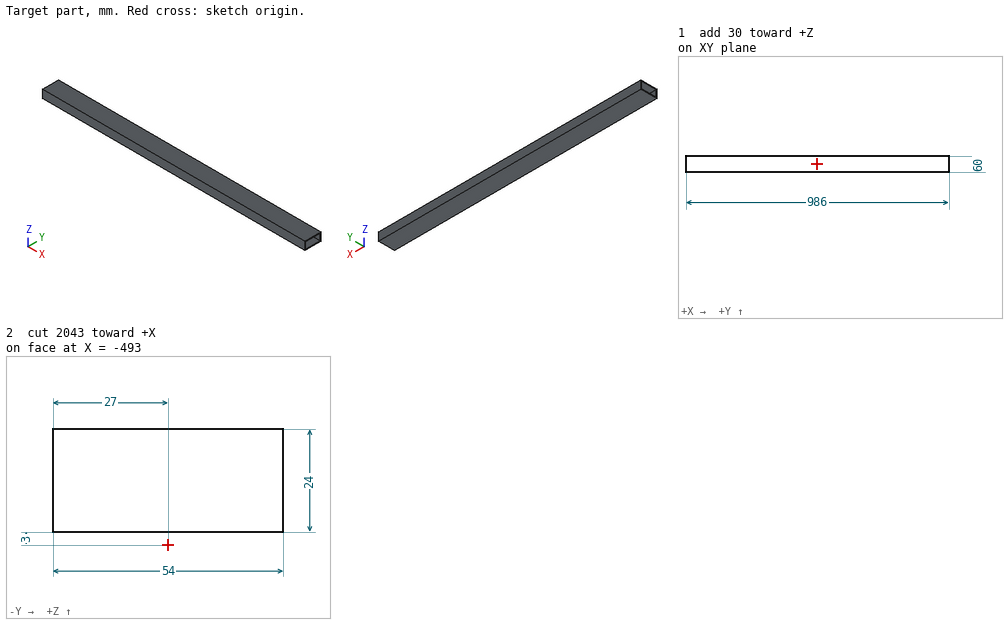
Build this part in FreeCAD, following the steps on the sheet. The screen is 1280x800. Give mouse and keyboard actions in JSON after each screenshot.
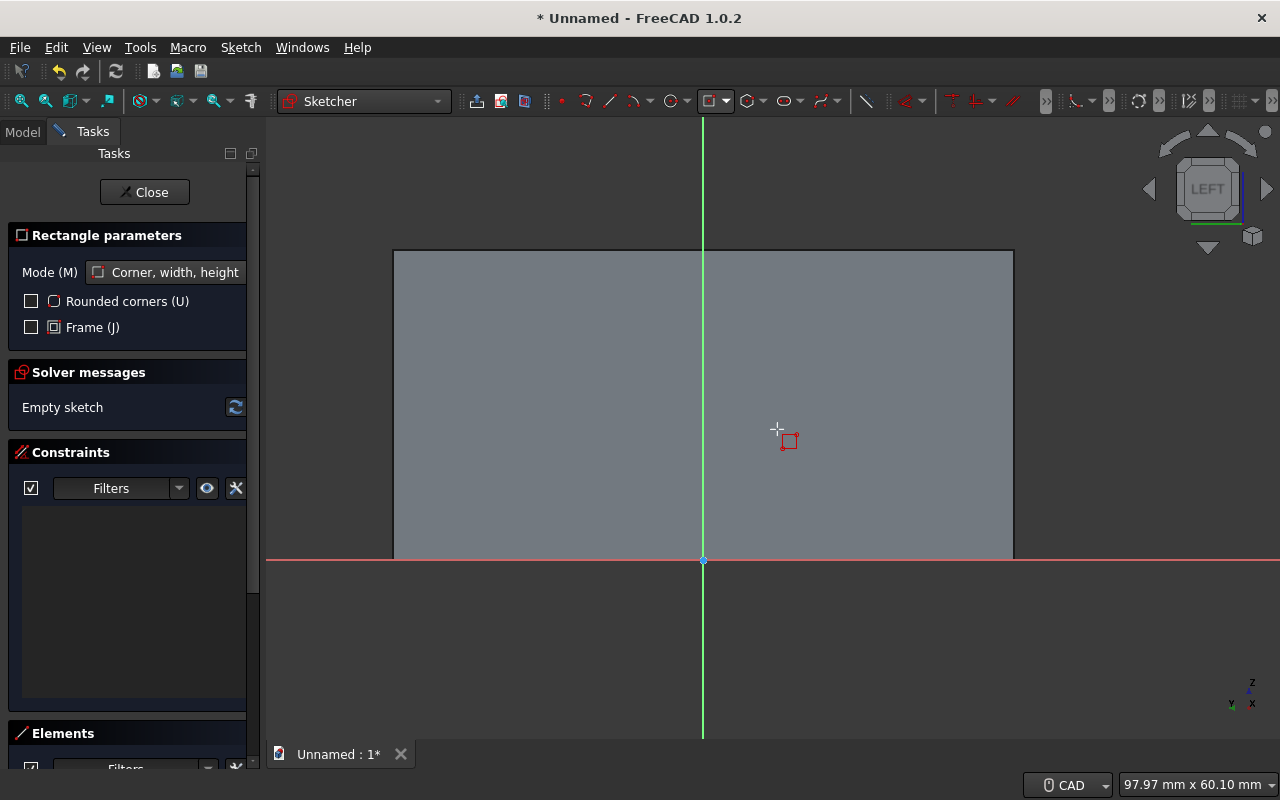
{"action": "left_click", "coordinate": [424, 281]}
{"action": "mouse_move", "coordinate": [983, 529]}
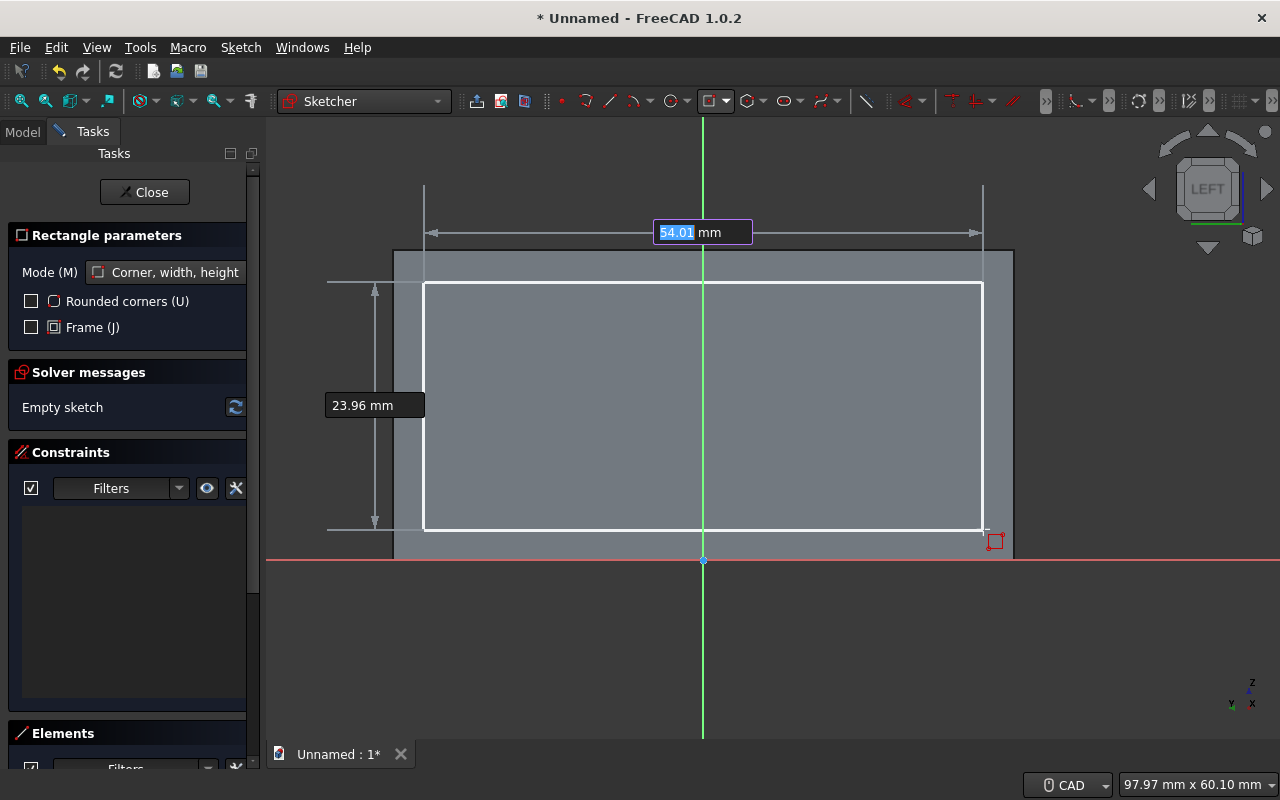
{"action": "type", "text": "54"}
{"action": "key", "text": "Tab"}
{"action": "type", "text": "24"}
{"action": "key", "text": "Return"}
{"action": "key", "text": "Escape"}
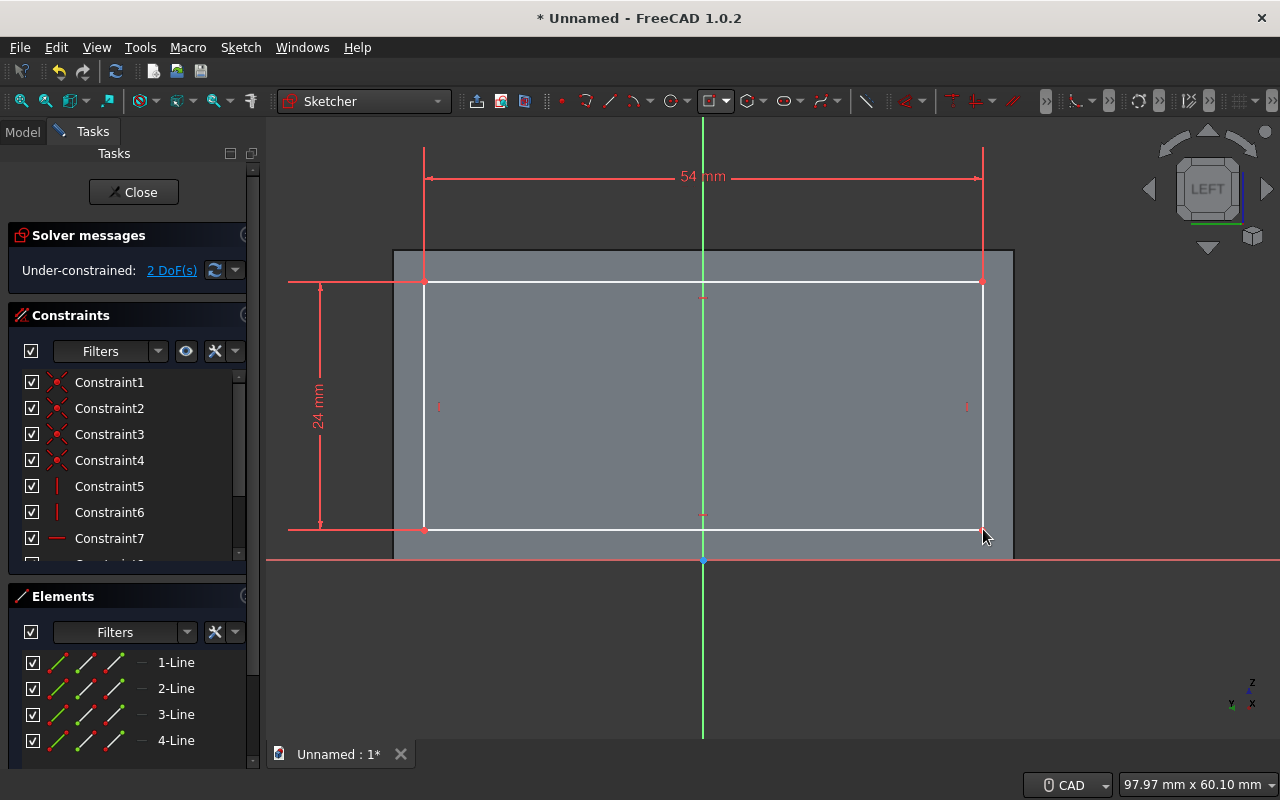
{"action": "scroll", "coordinate": [424, 530], "scroll_direction": "up", "scroll_amount": 2}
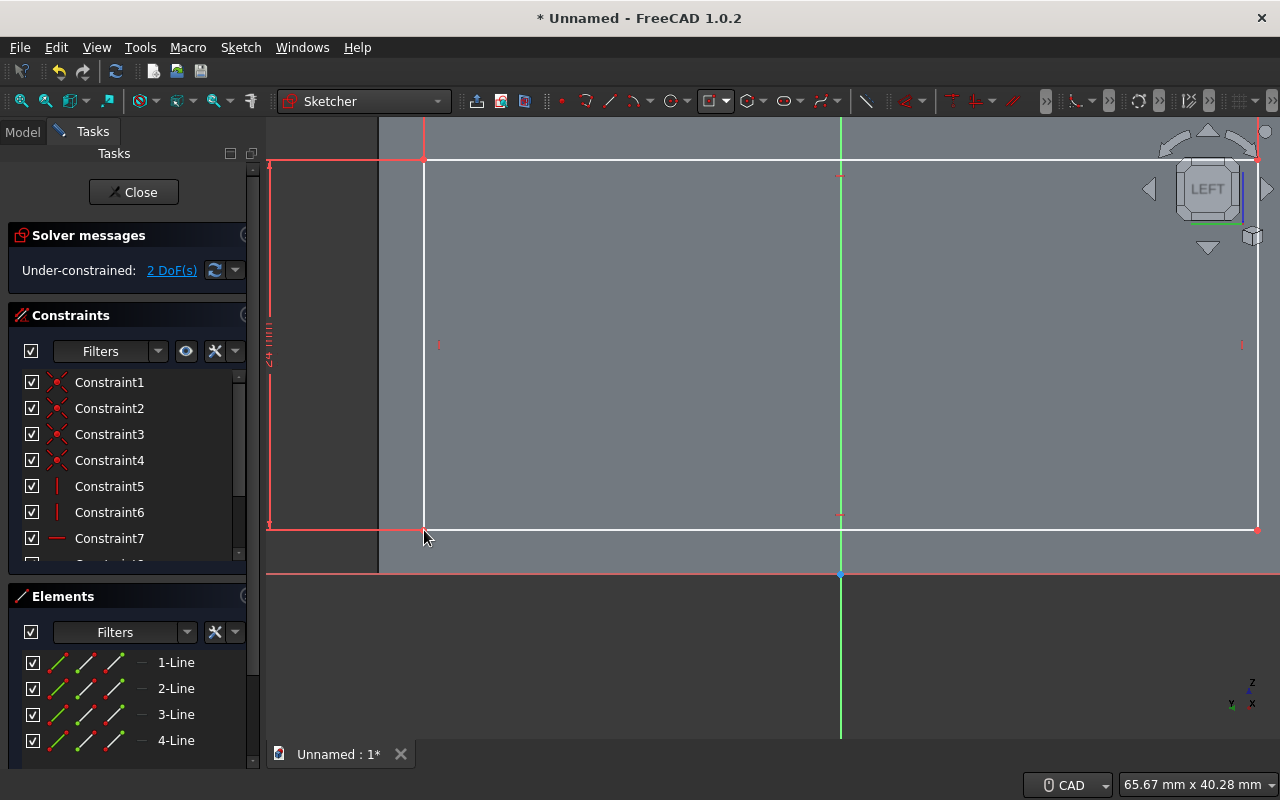
{"action": "left_click", "coordinate": [424, 530]}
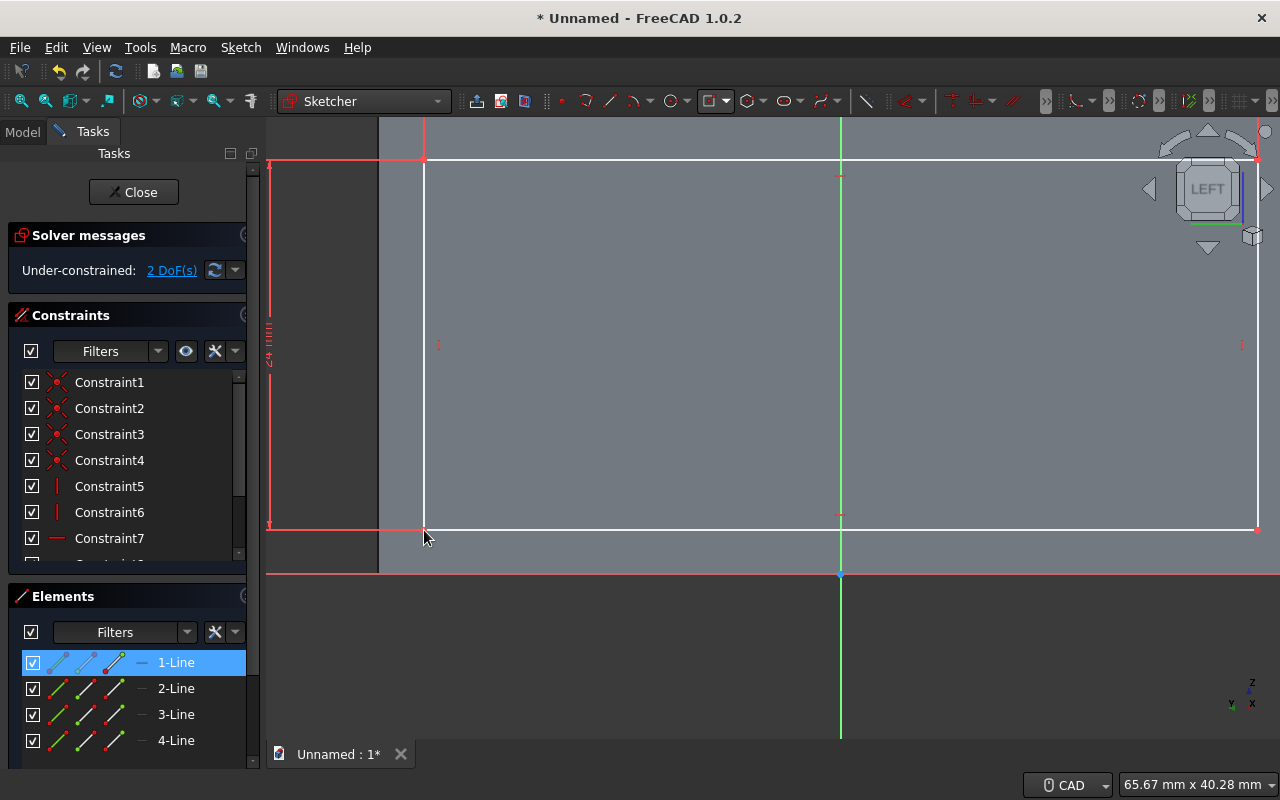
{"action": "key", "text": "i"}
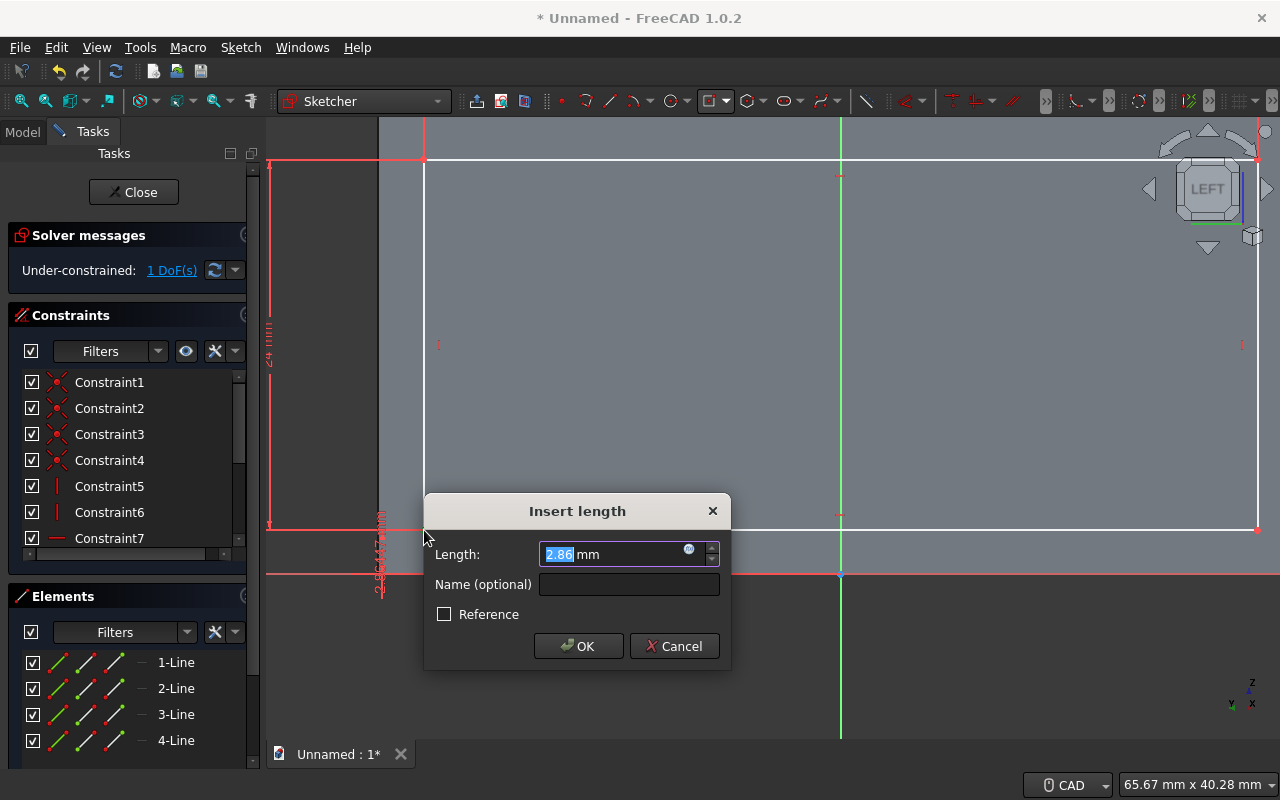
{"action": "type", "text": "3"}
{"action": "key", "text": "Return"}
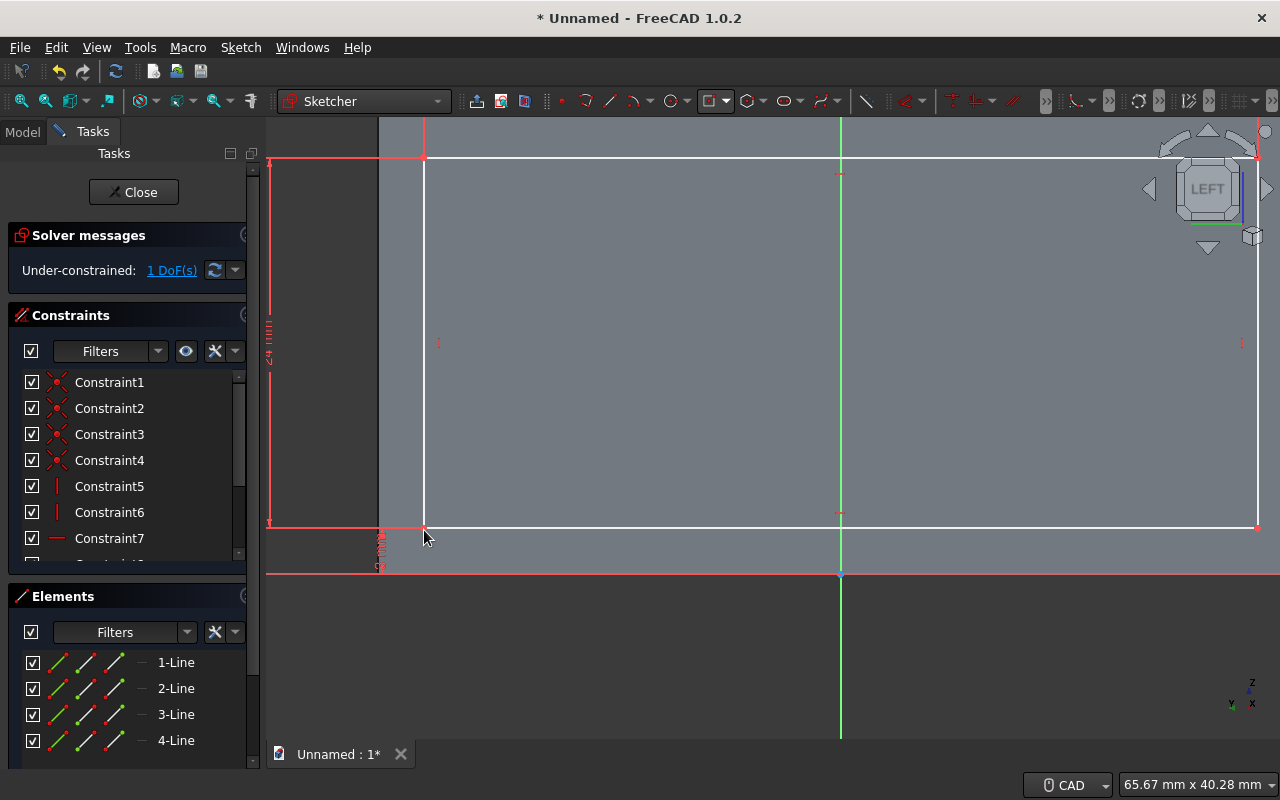
{"action": "left_click", "coordinate": [424, 158]}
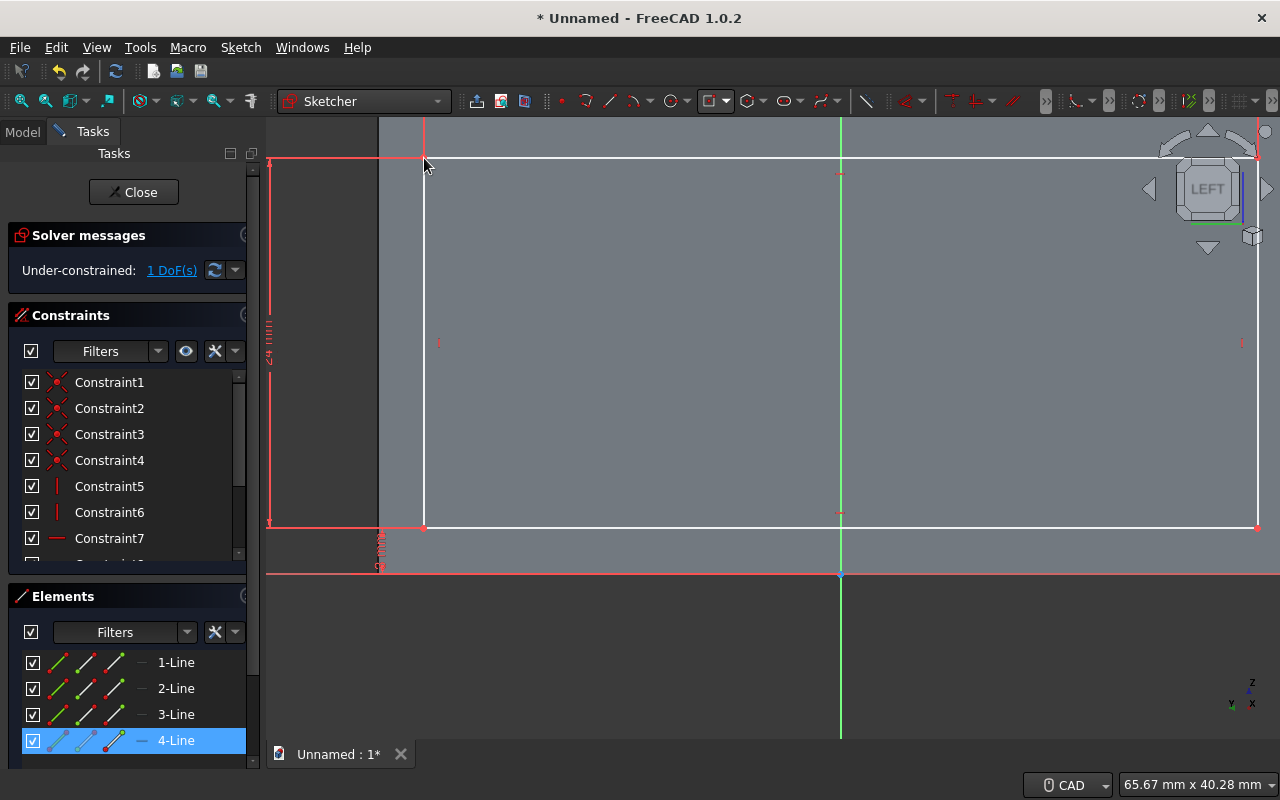
{"action": "left_click", "coordinate": [924, 102]}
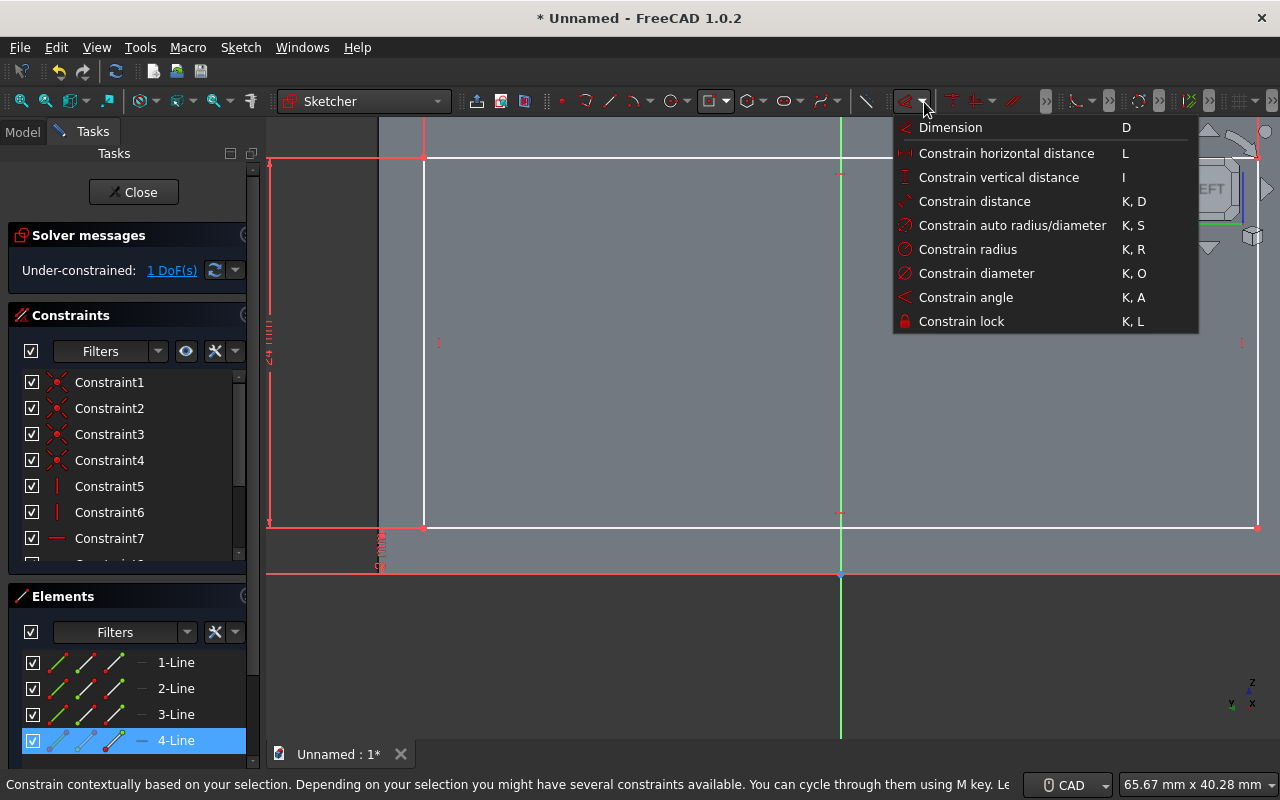
{"action": "left_click", "coordinate": [1046, 153]}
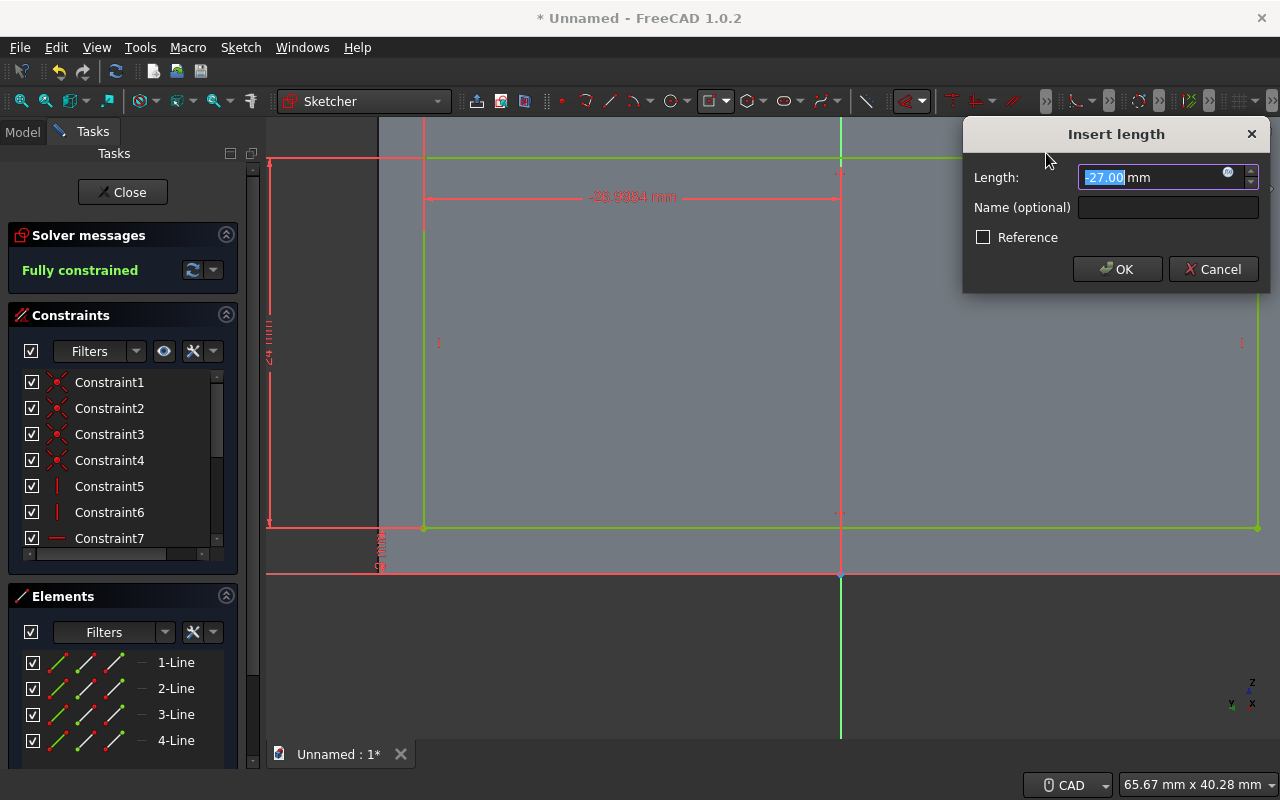
{"action": "type", "text": "-27"}
{"action": "key", "text": "Return"}